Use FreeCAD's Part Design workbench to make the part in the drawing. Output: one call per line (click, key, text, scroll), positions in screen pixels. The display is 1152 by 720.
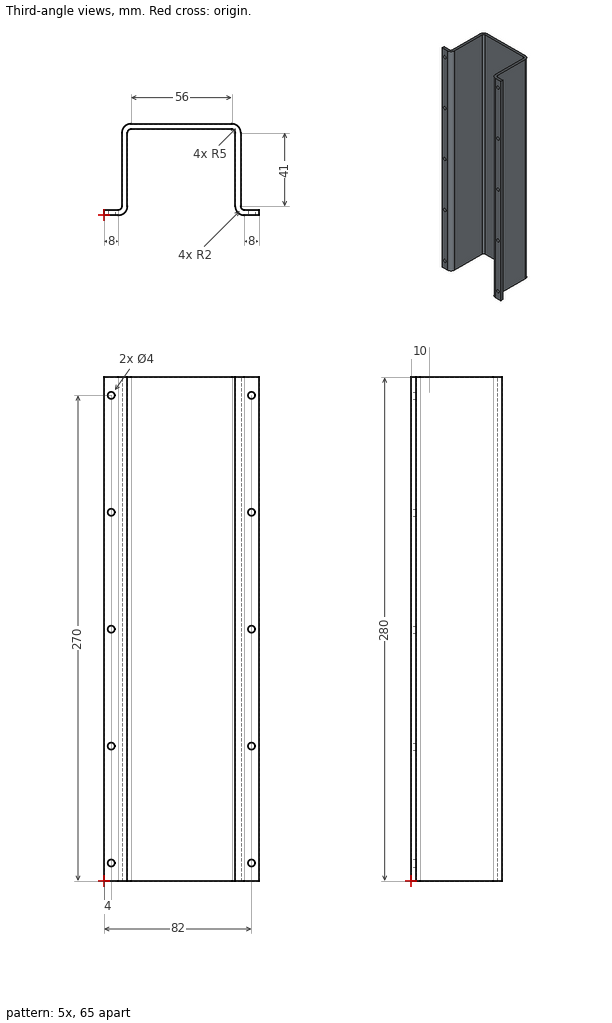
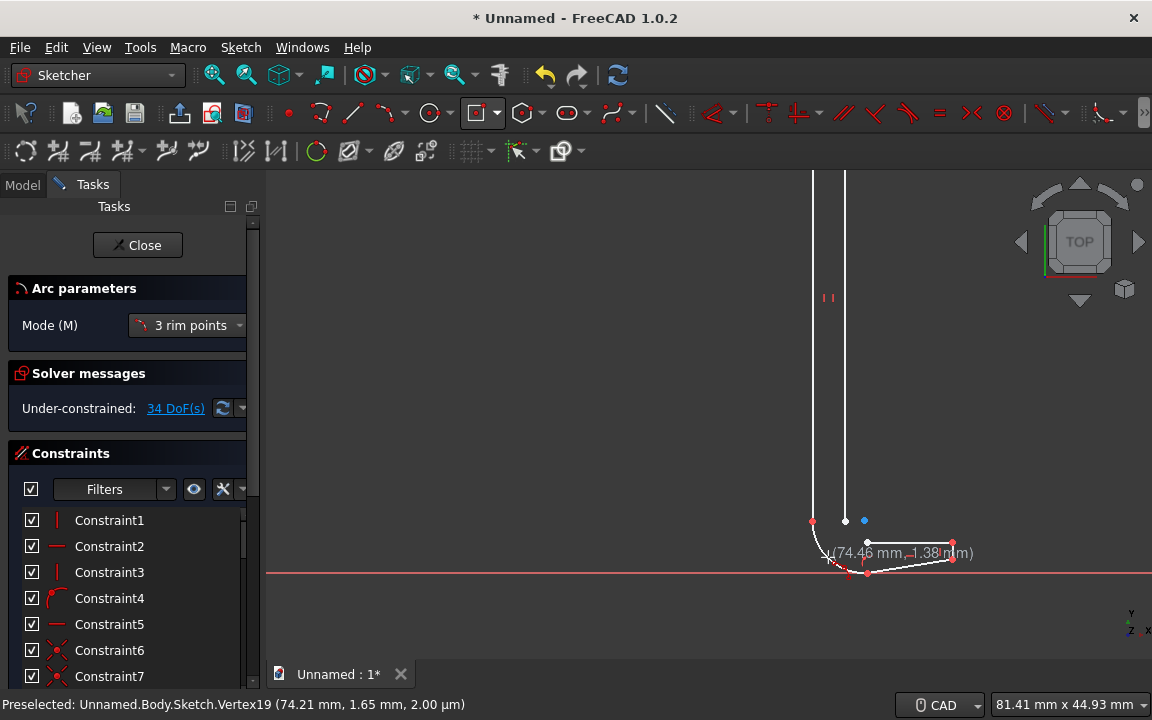
click(867, 543)
click(845, 521)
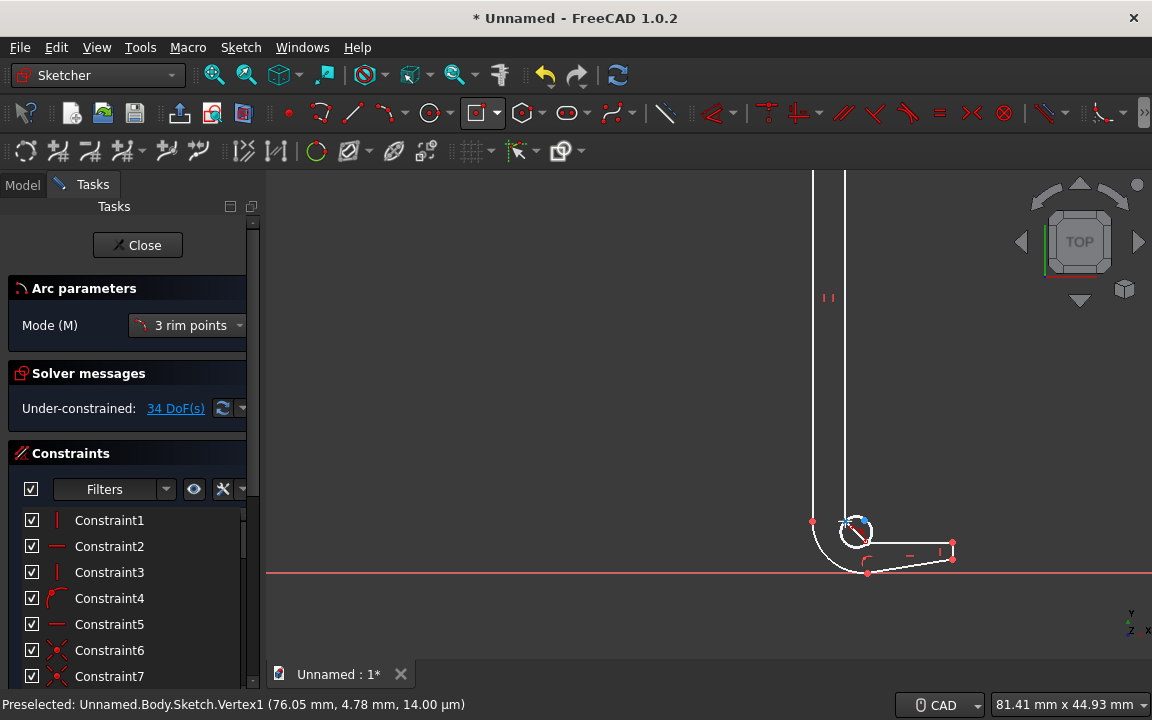
scroll(851, 534, up, 5)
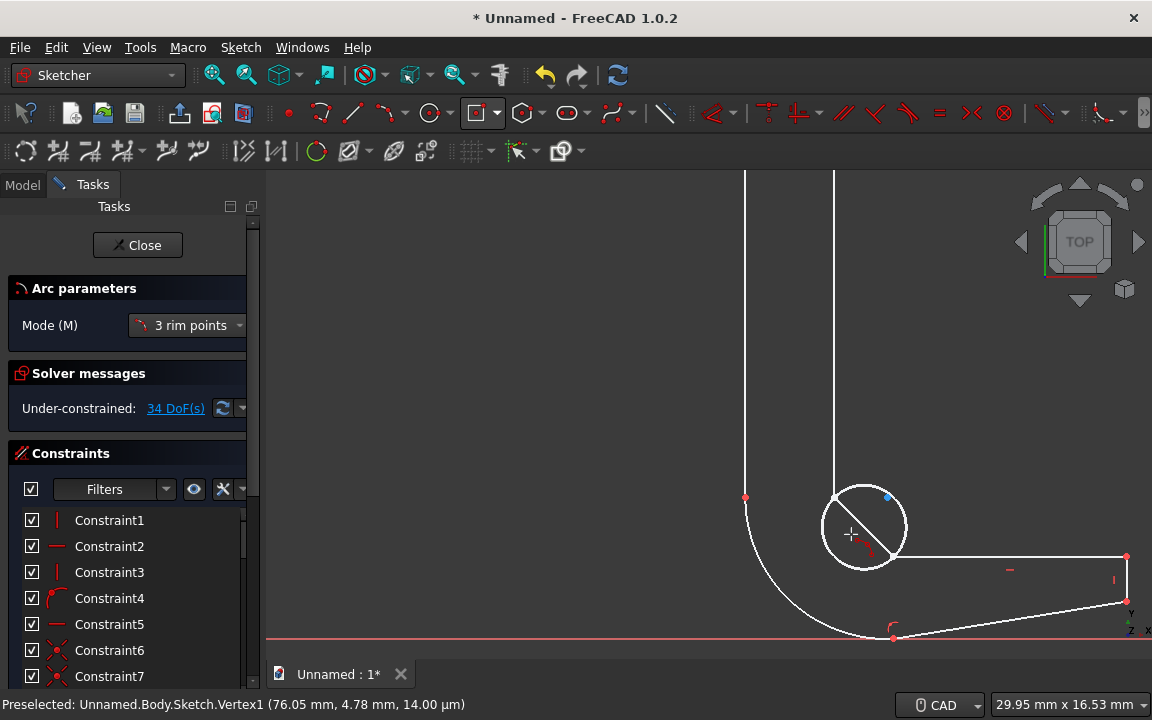
click(850, 533)
key(Escape)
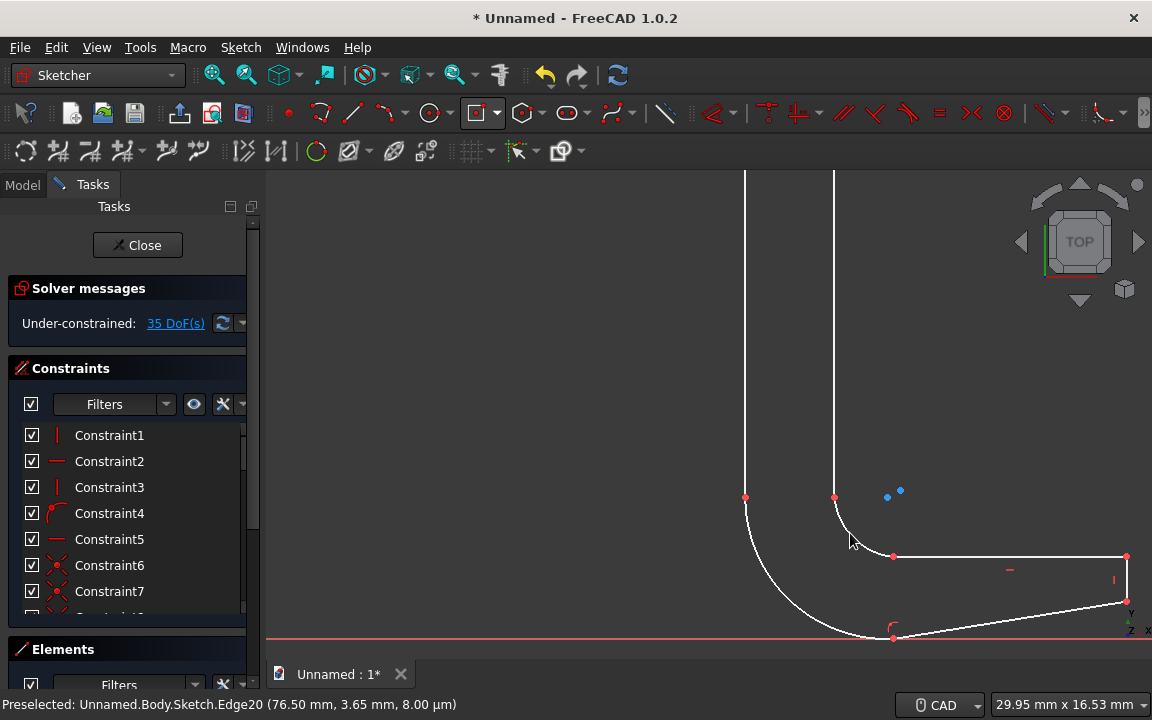
scroll(839, 549, down, 8)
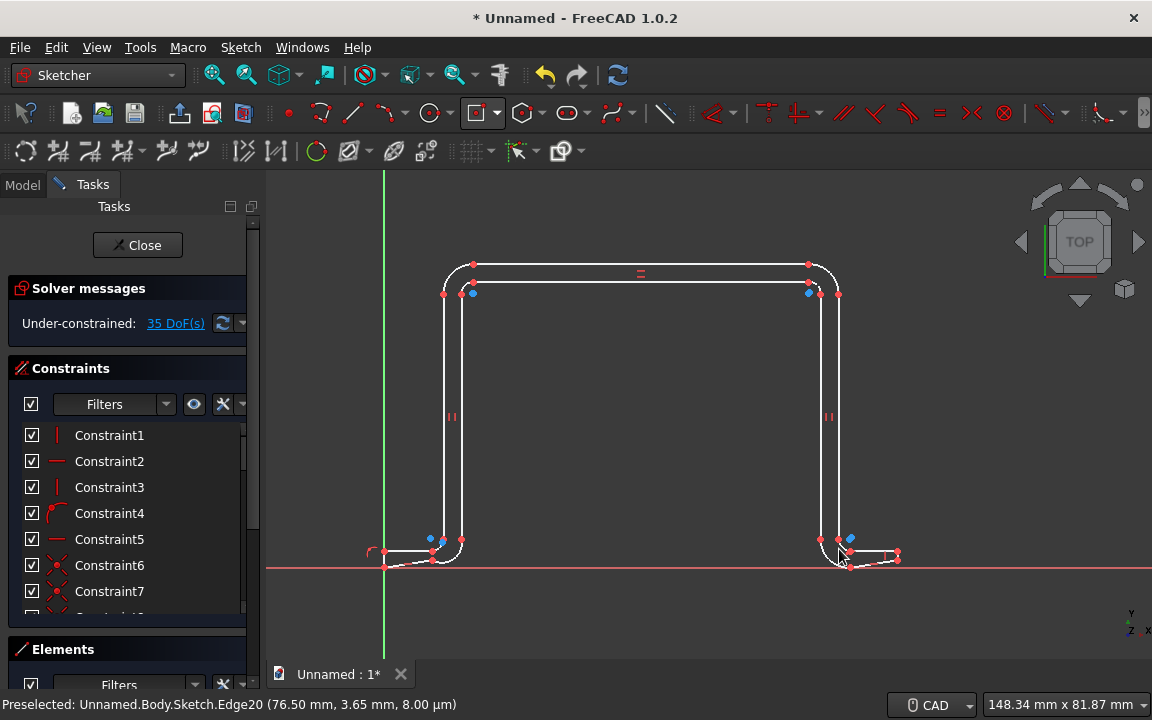
click(839, 490)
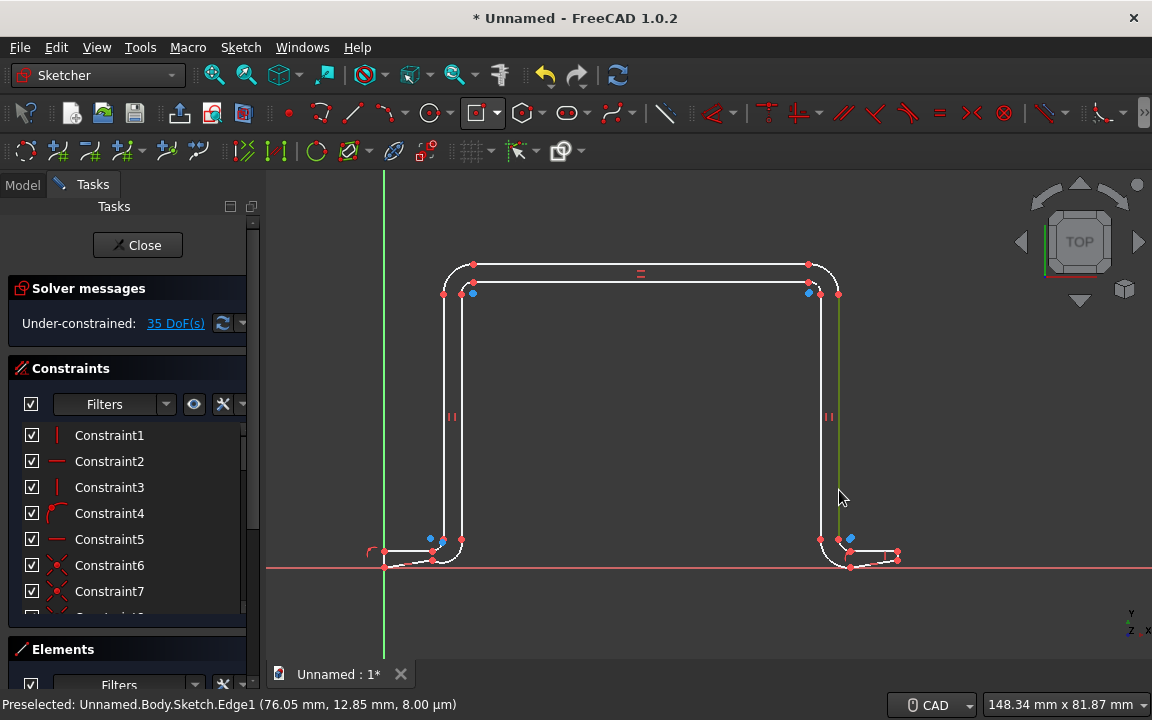
click(835, 281)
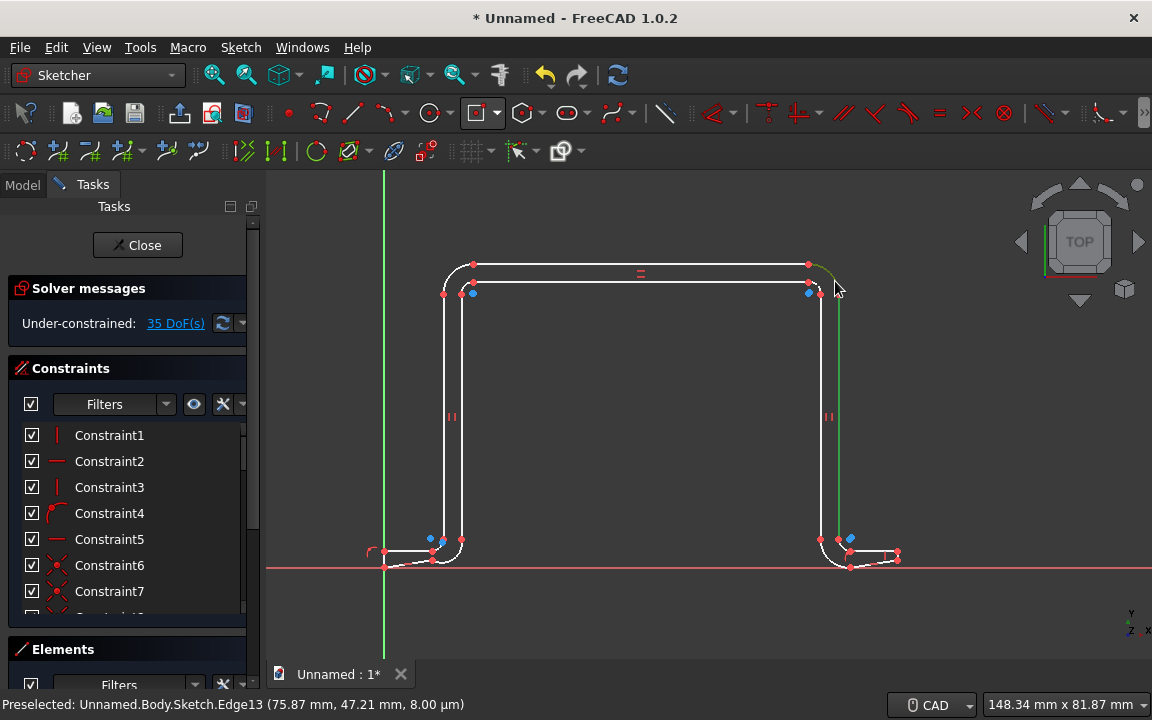
key(t)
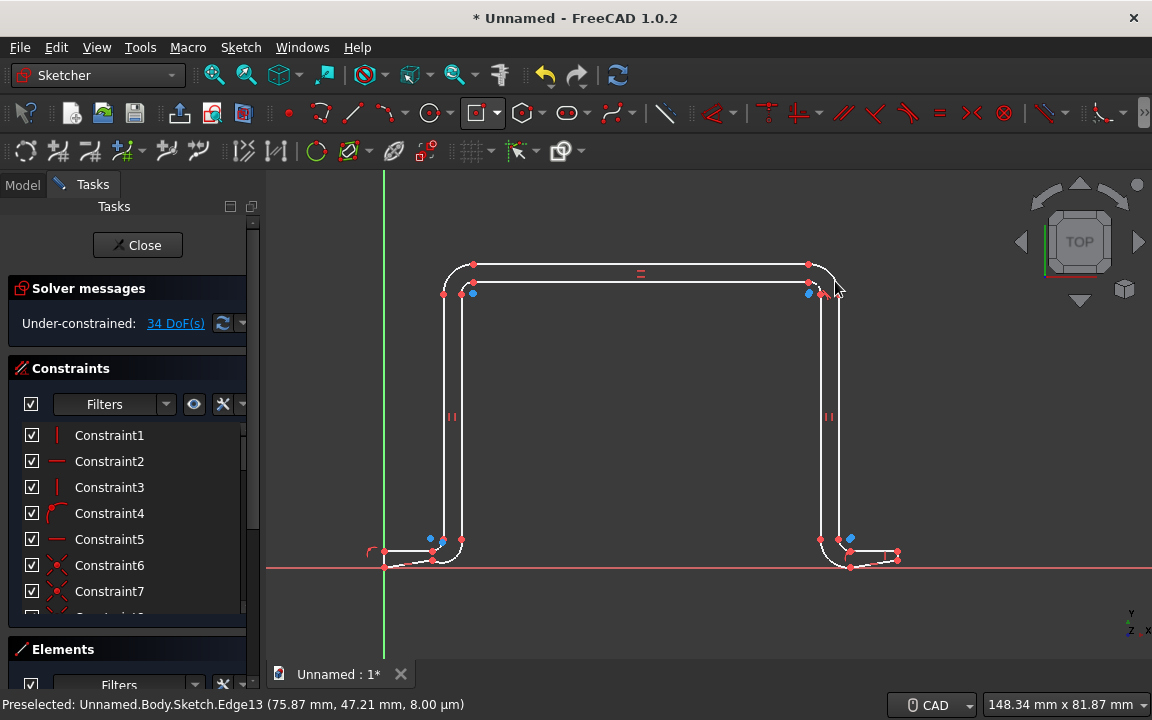
click(839, 466)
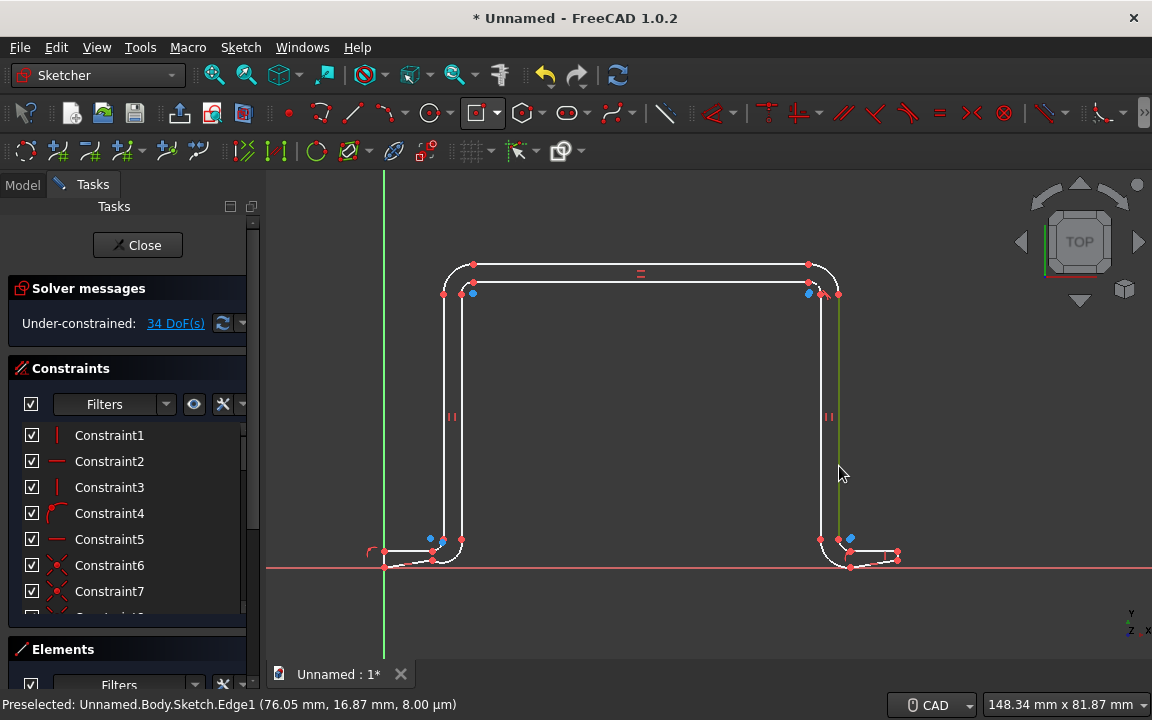
scroll(842, 547, up, 3)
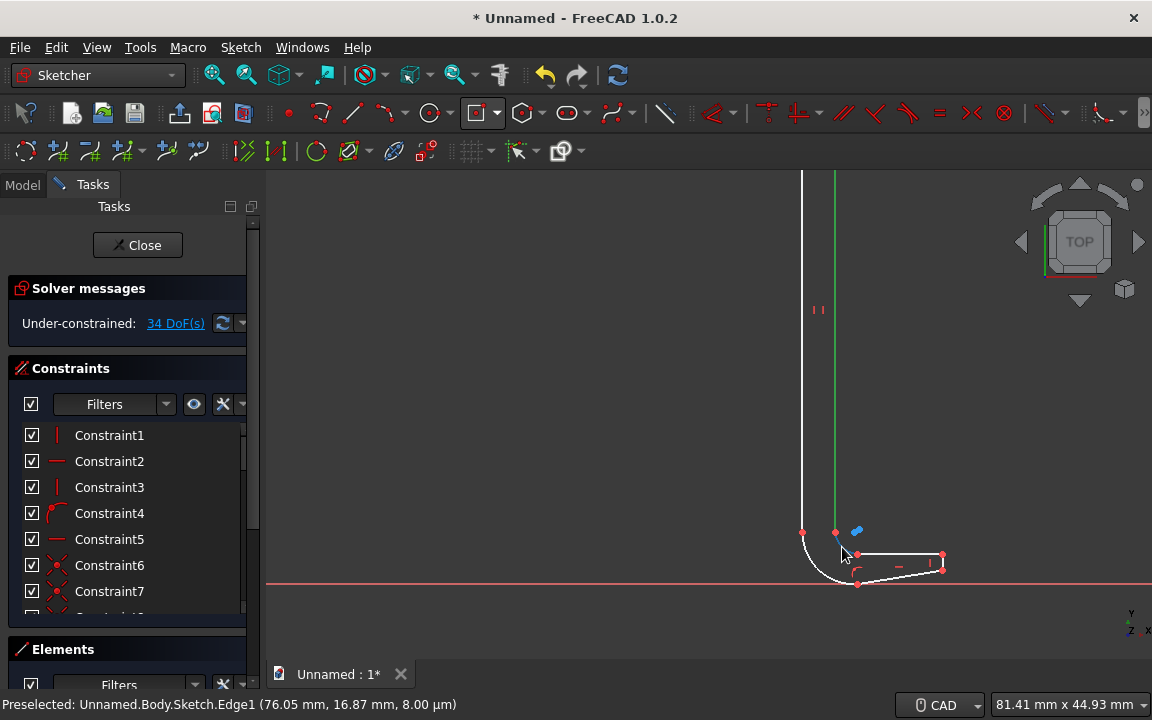
click(842, 547)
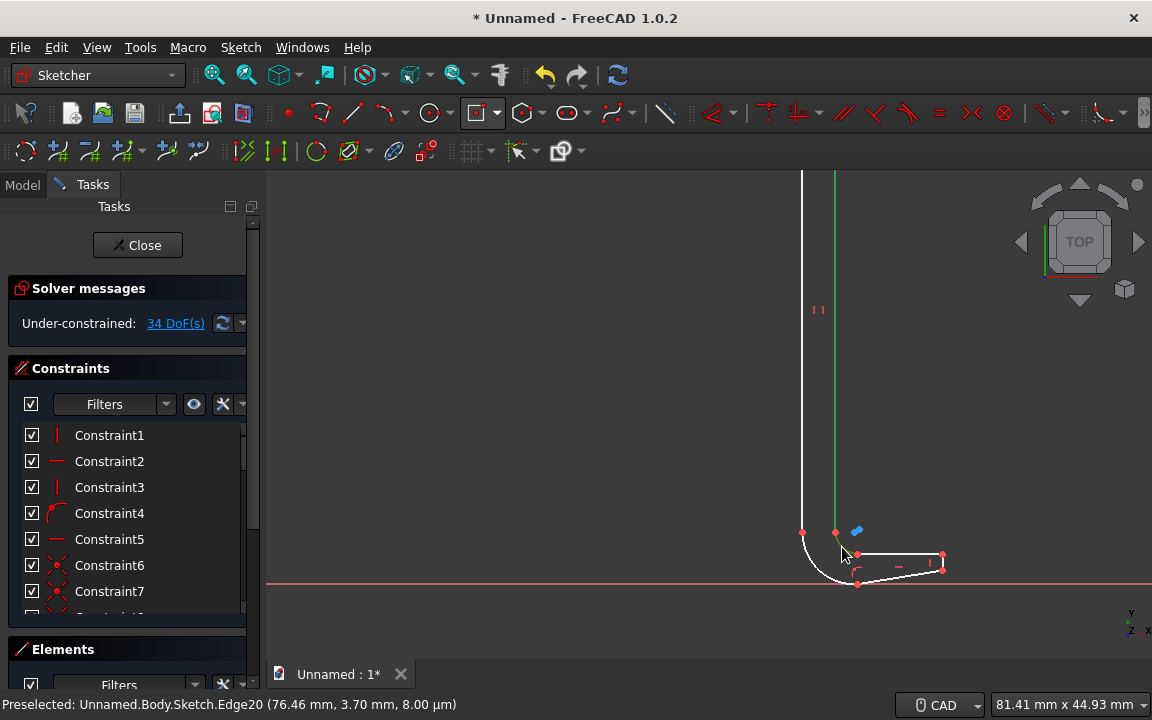
click(908, 114)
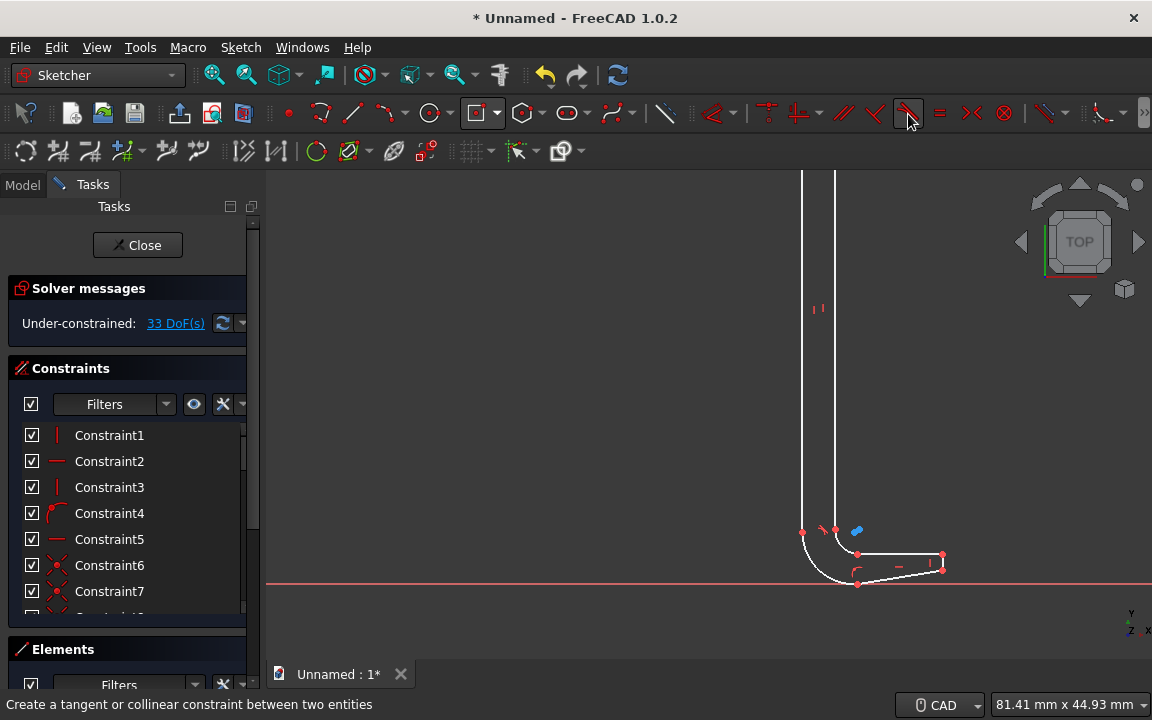
scroll(841, 546, down, 3)